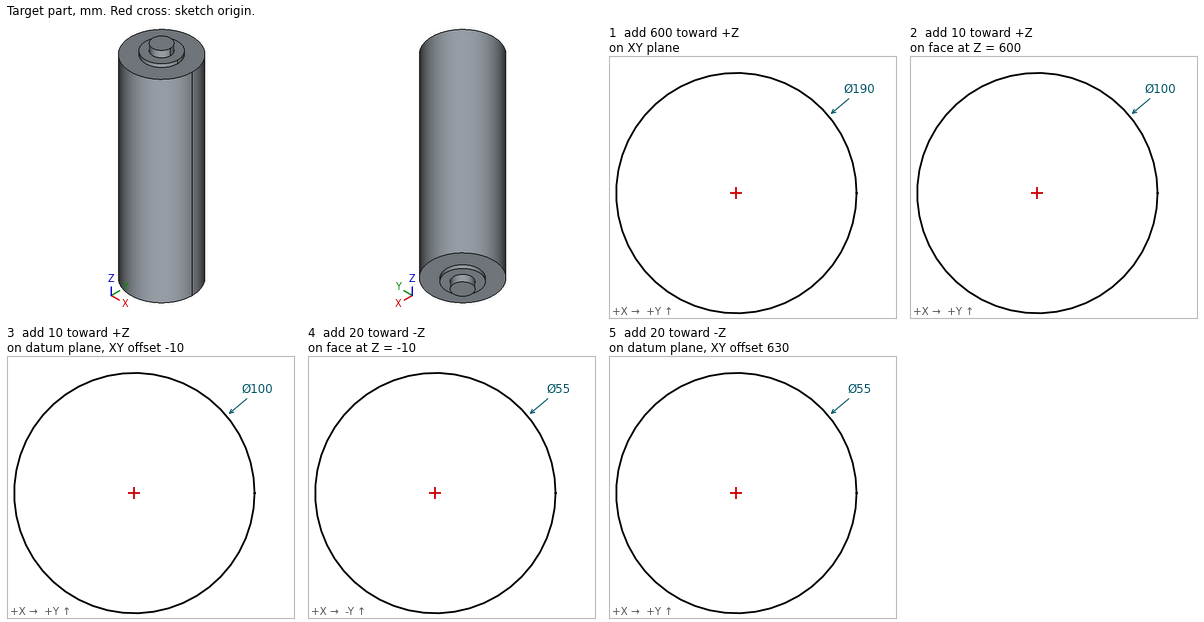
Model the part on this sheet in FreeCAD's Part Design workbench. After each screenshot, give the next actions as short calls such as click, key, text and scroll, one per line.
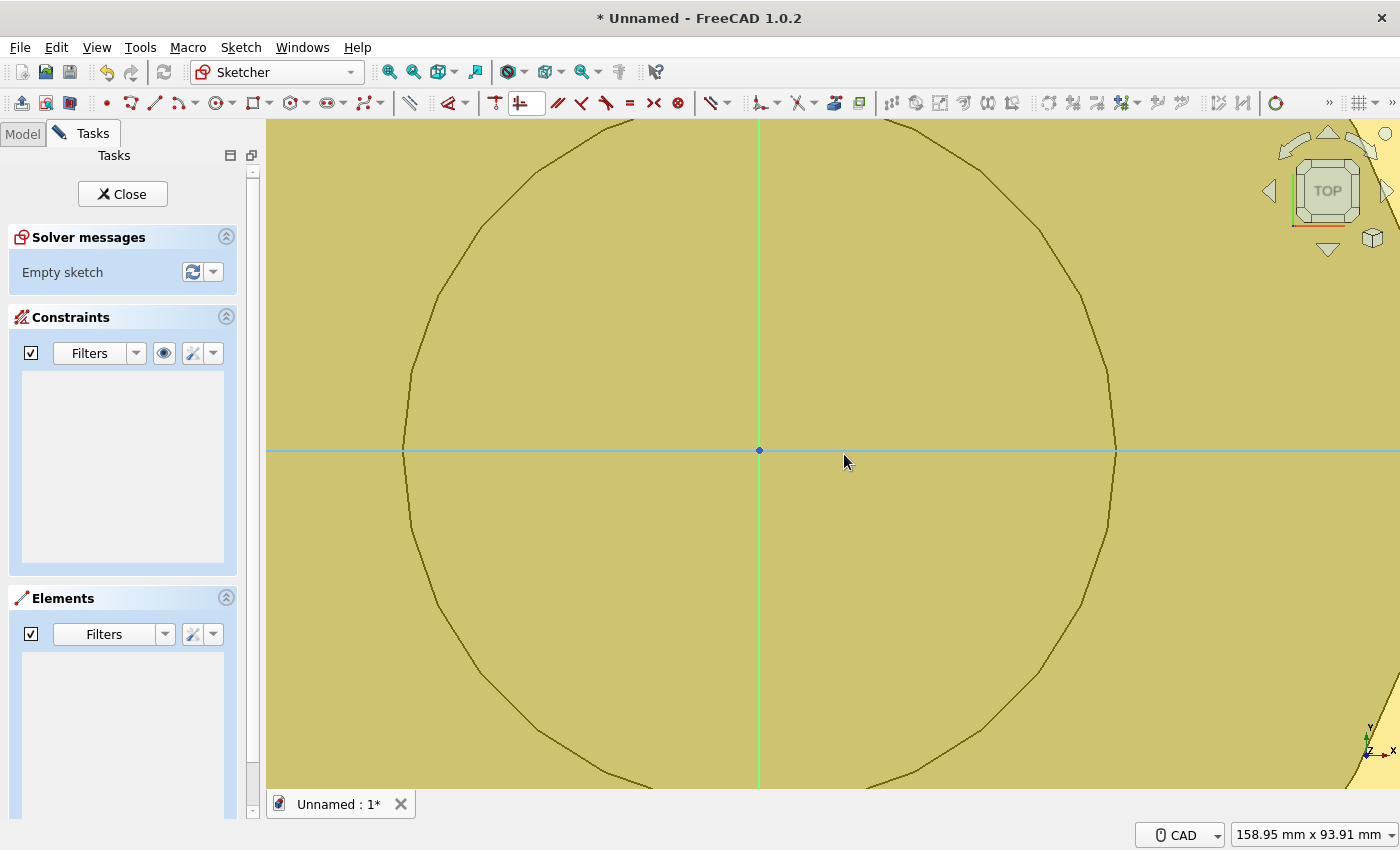
click(216, 104)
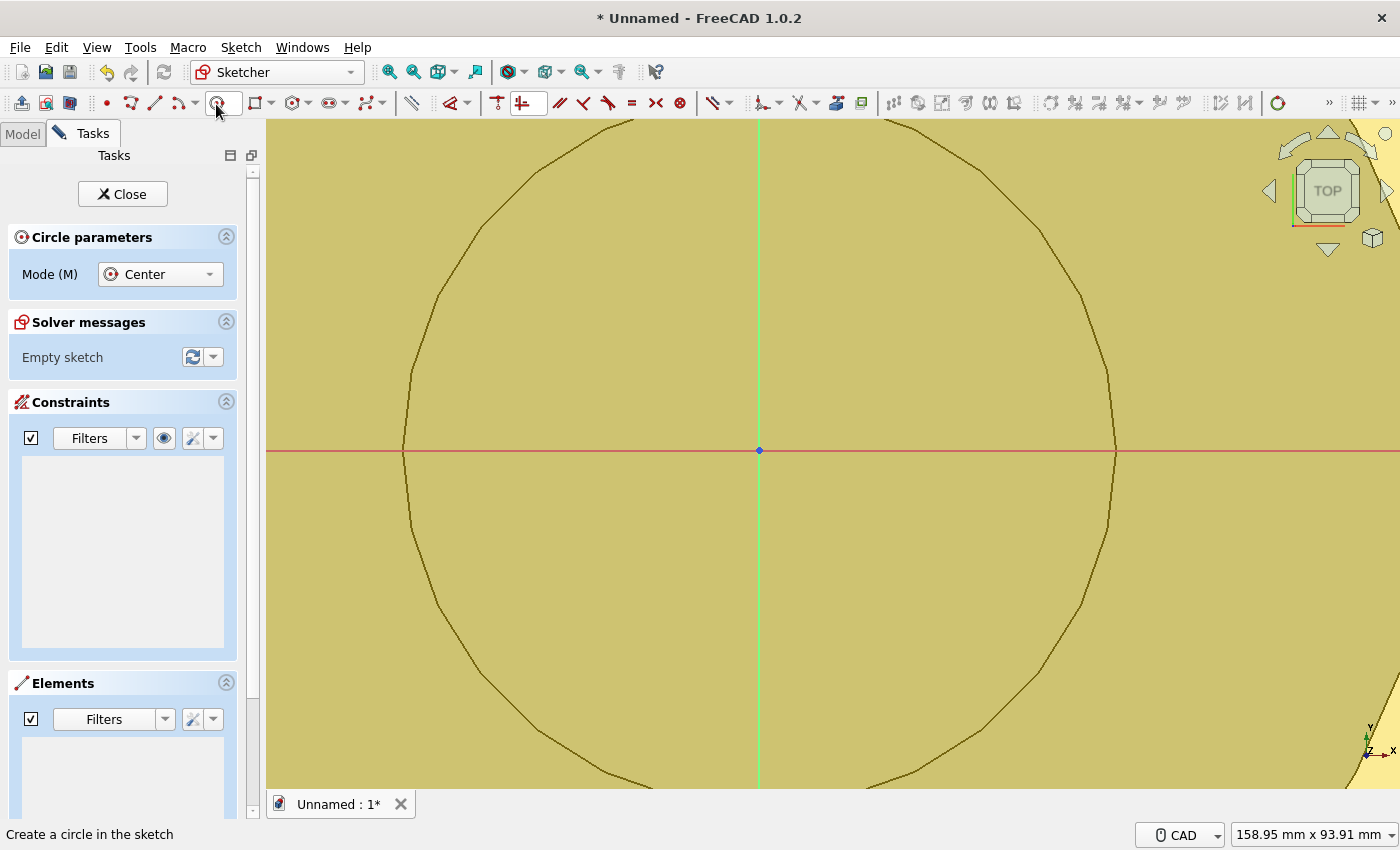
click(759, 451)
click(898, 312)
key(Escape)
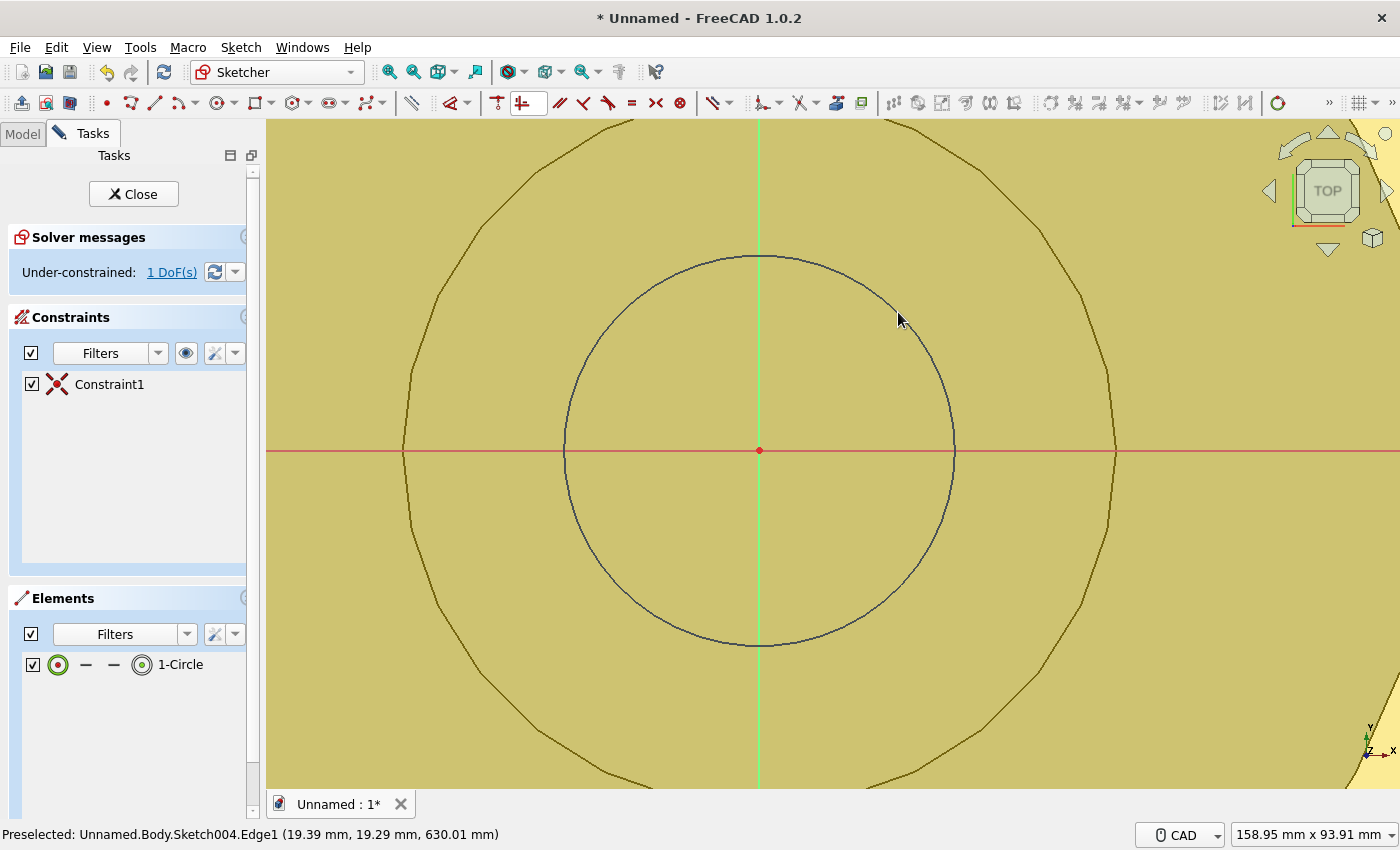
click(450, 104)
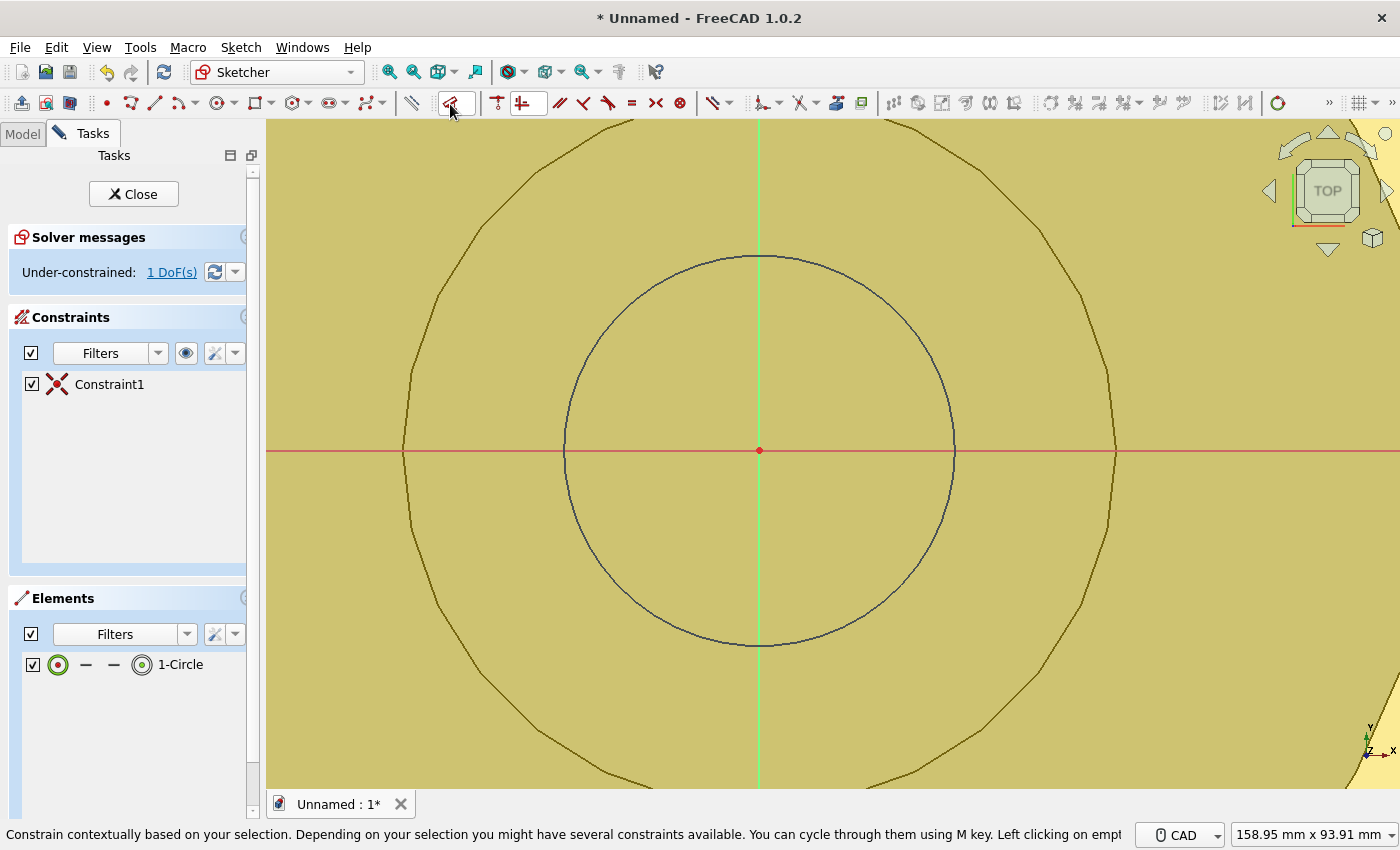
click(897, 312)
click(920, 289)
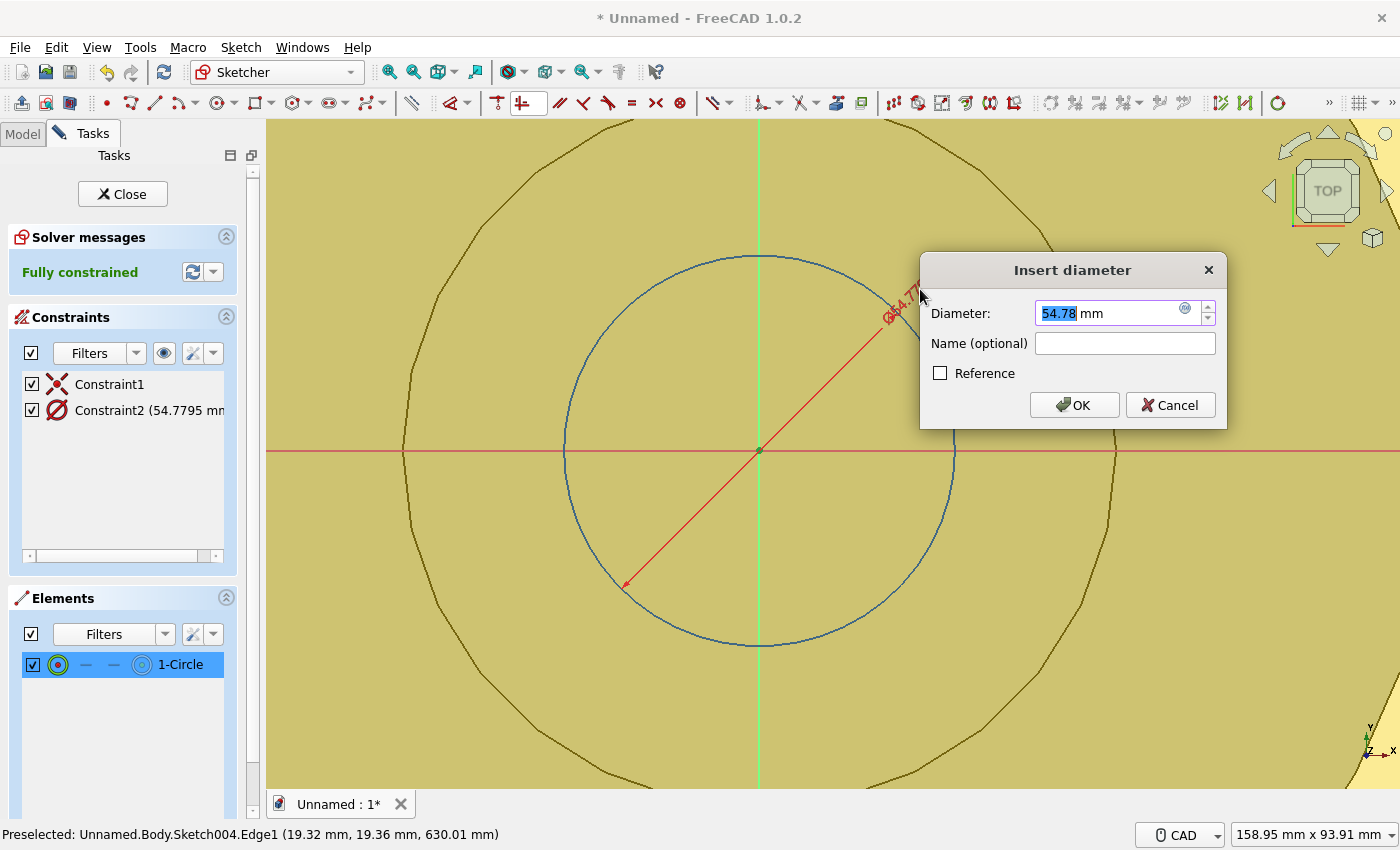
text(55)
key(Return)
key(Escape)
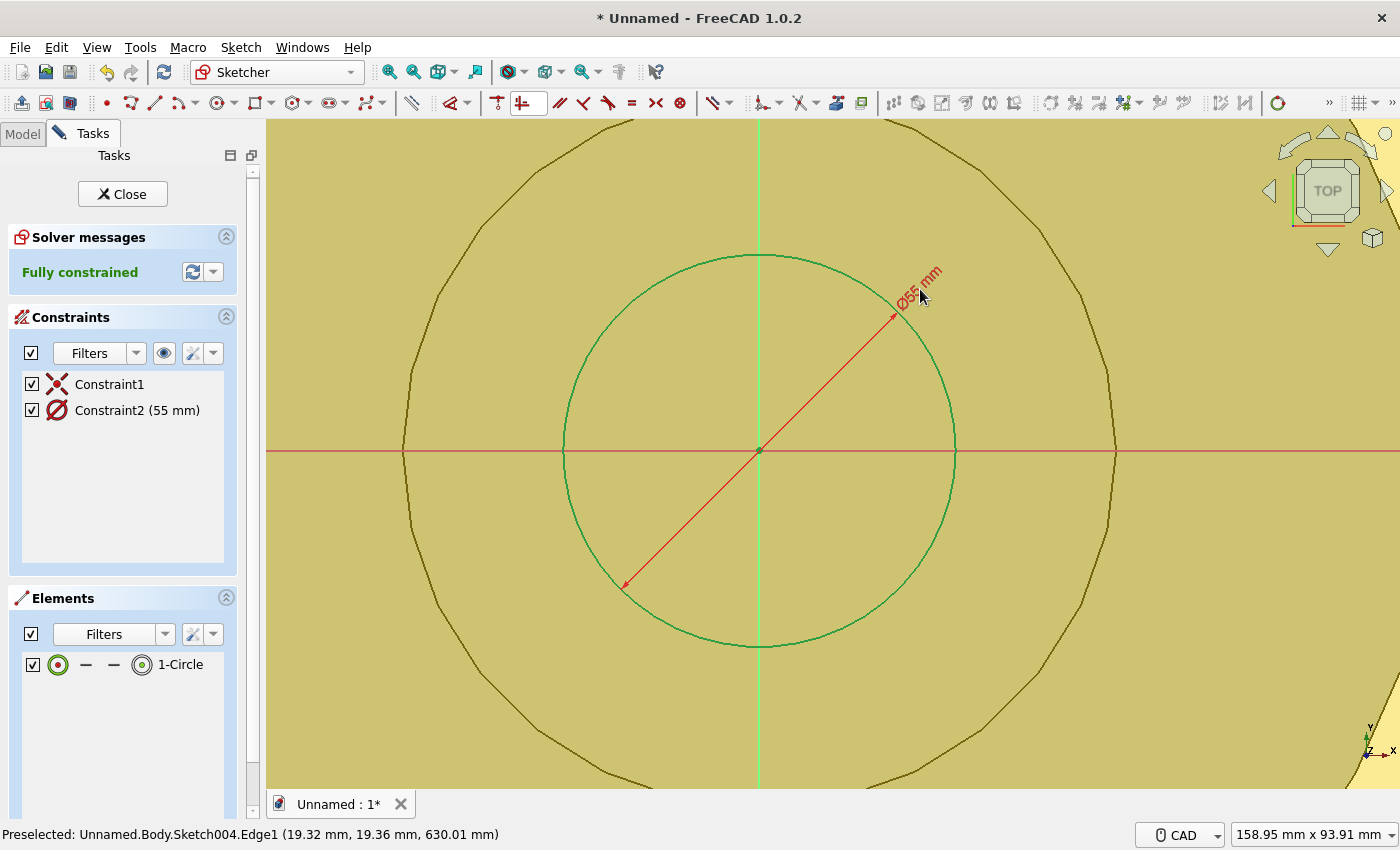
click(123, 194)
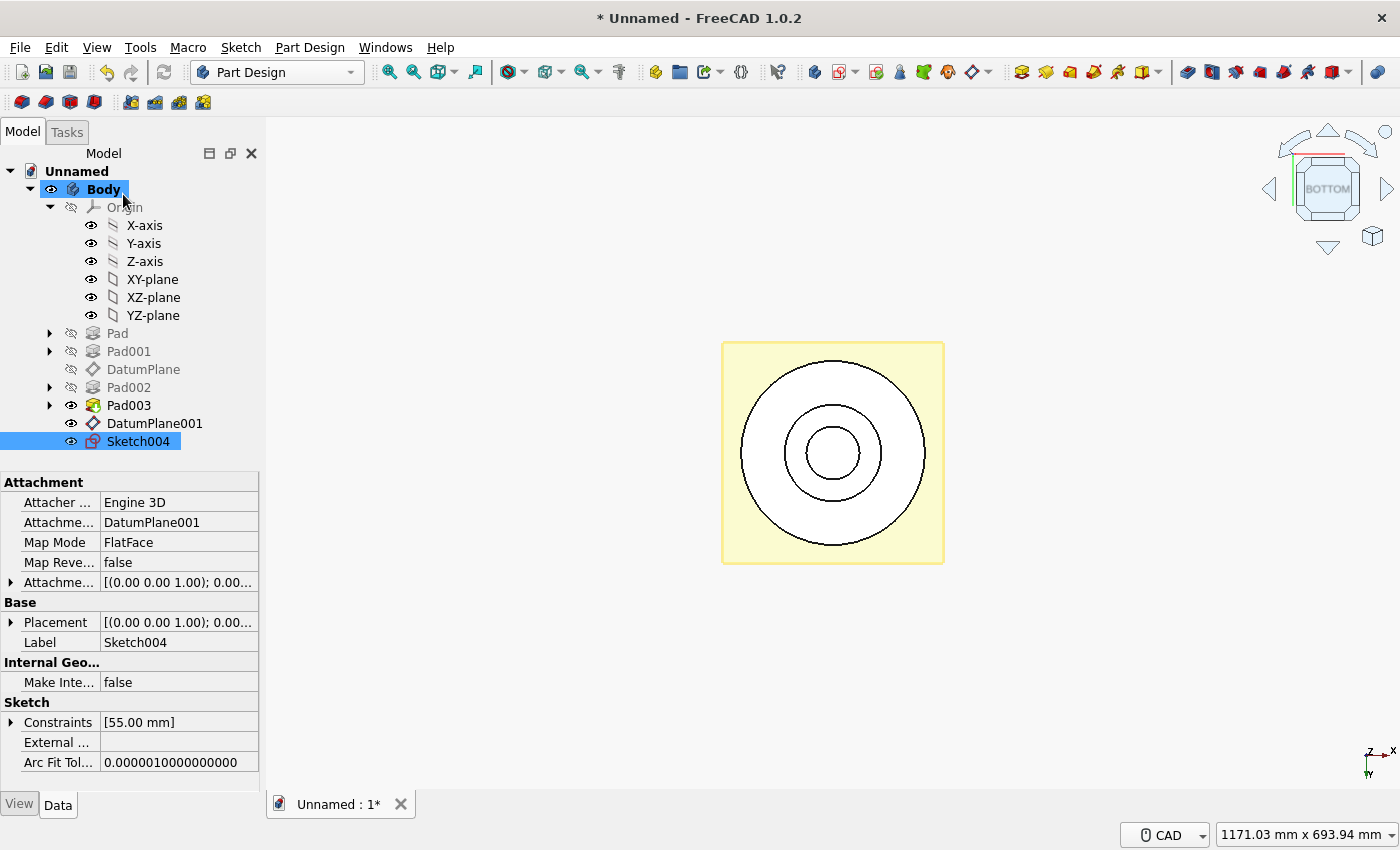
click(1022, 72)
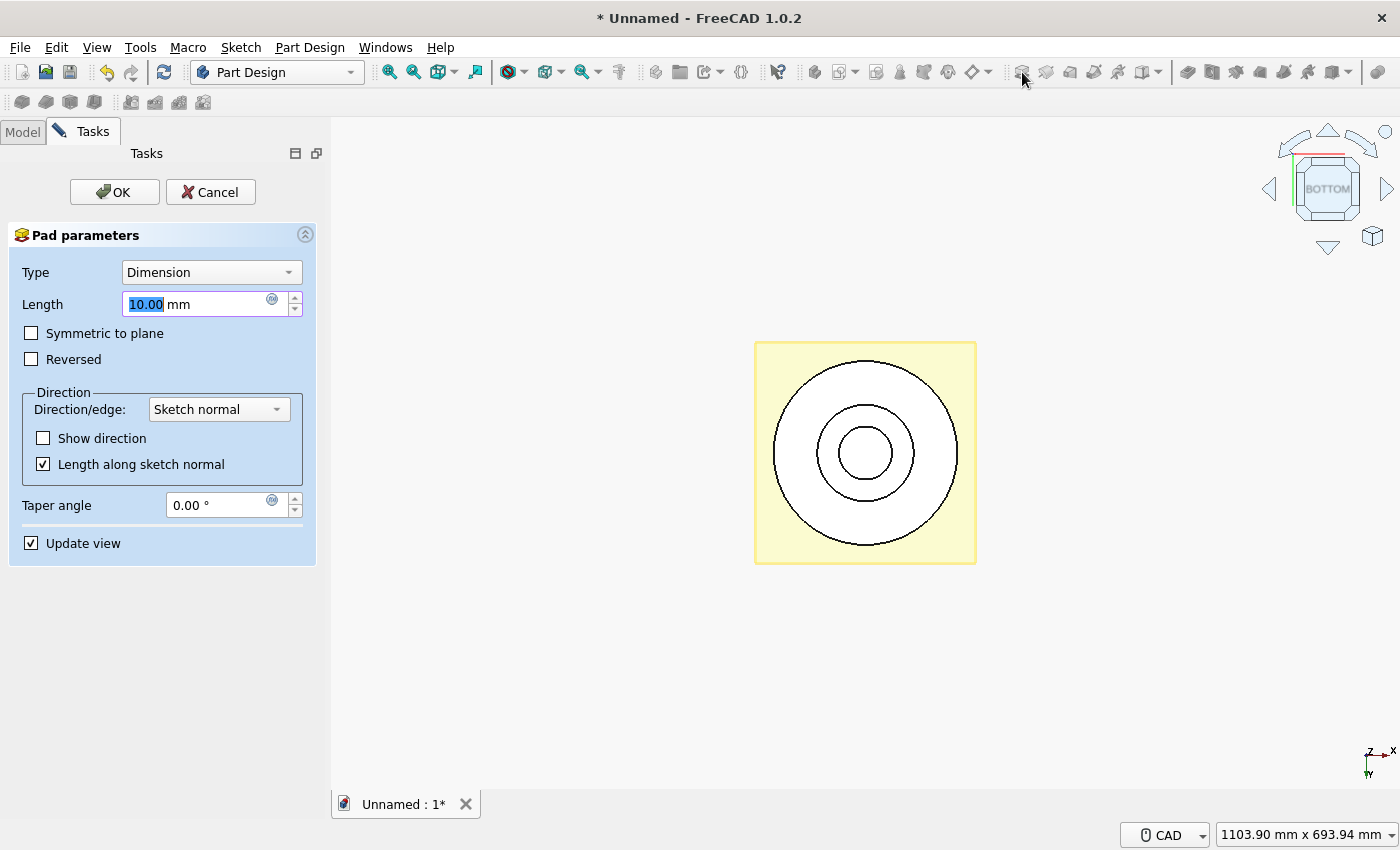
text(20)
key(Tab)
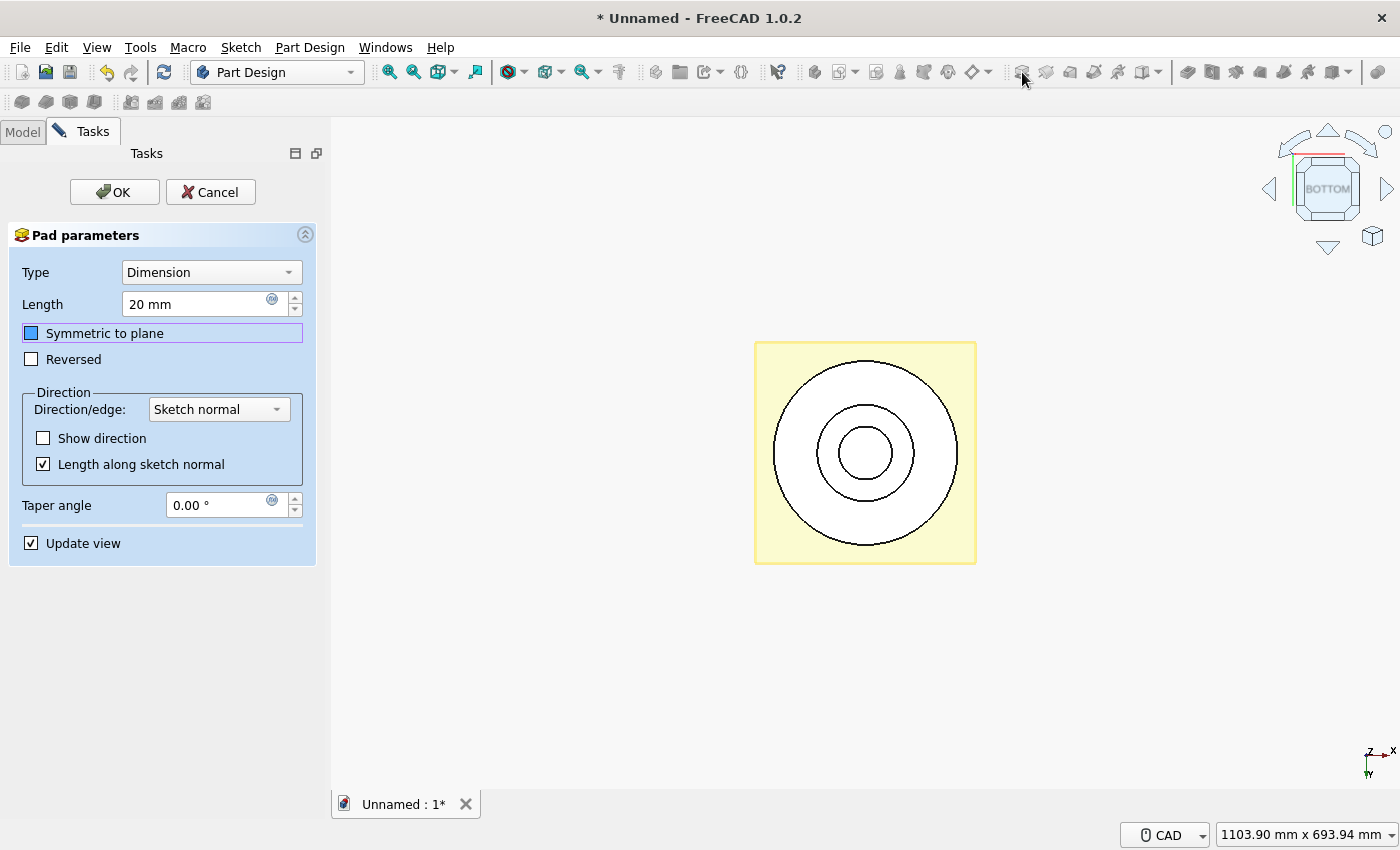
click(30, 359)